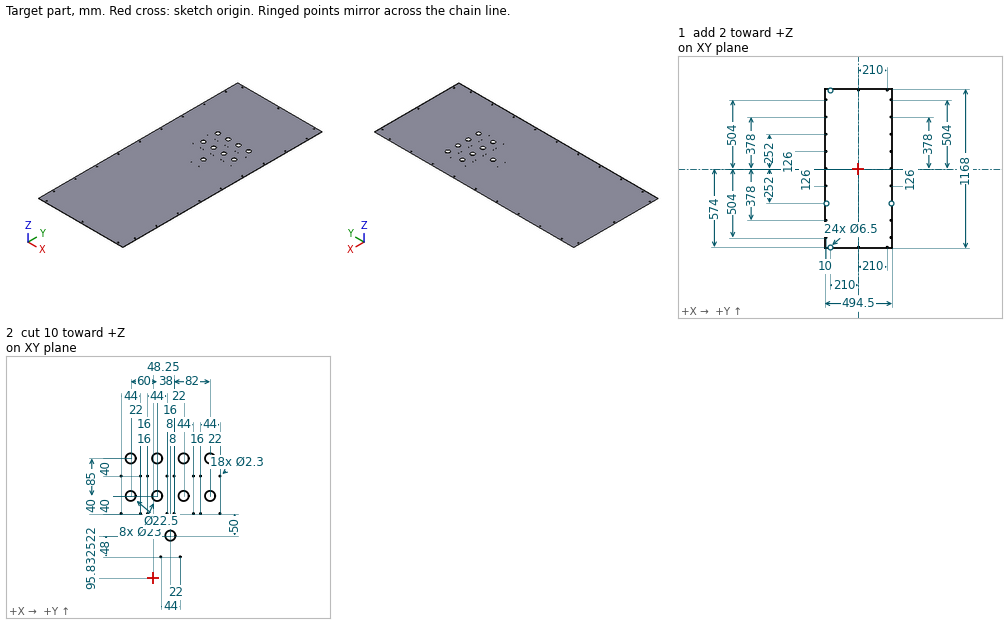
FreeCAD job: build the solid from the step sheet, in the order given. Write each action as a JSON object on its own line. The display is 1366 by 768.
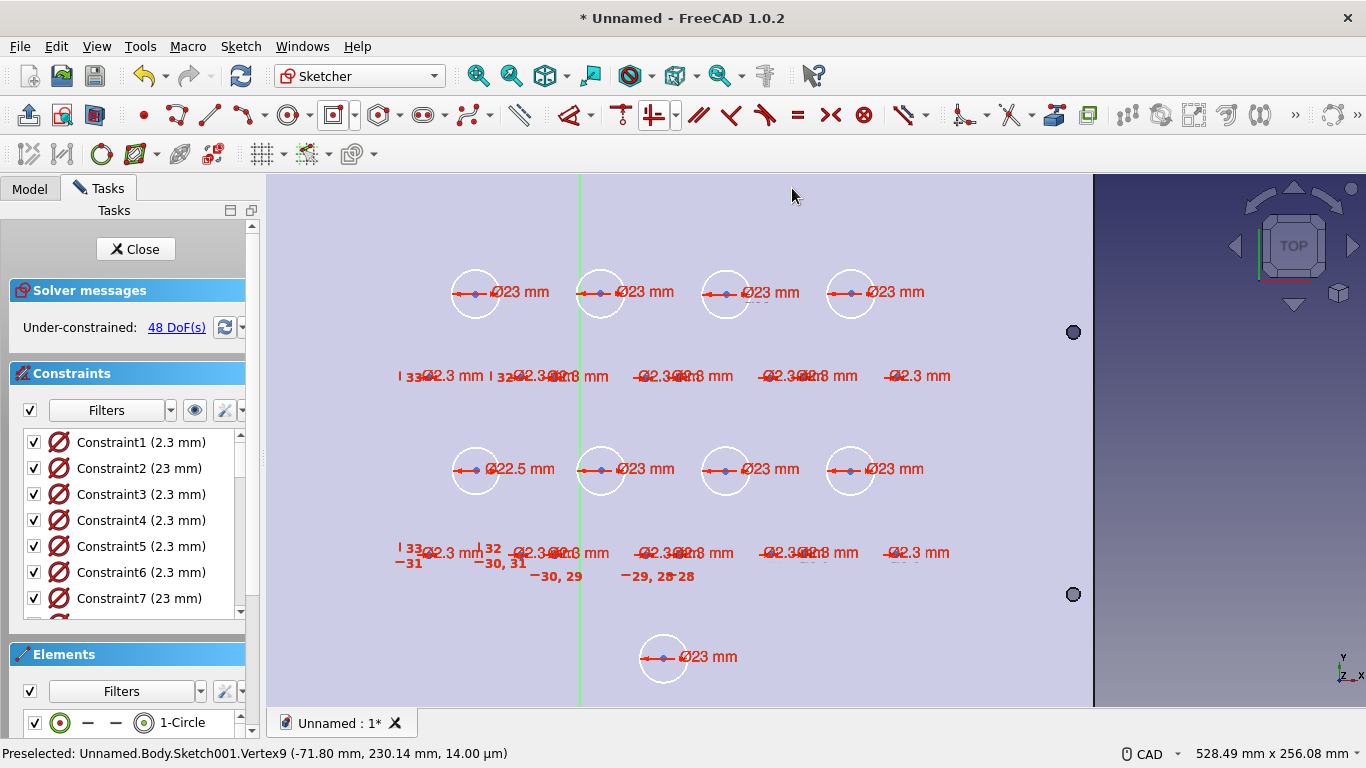
{"action": "left_click", "coordinate": [521, 378]}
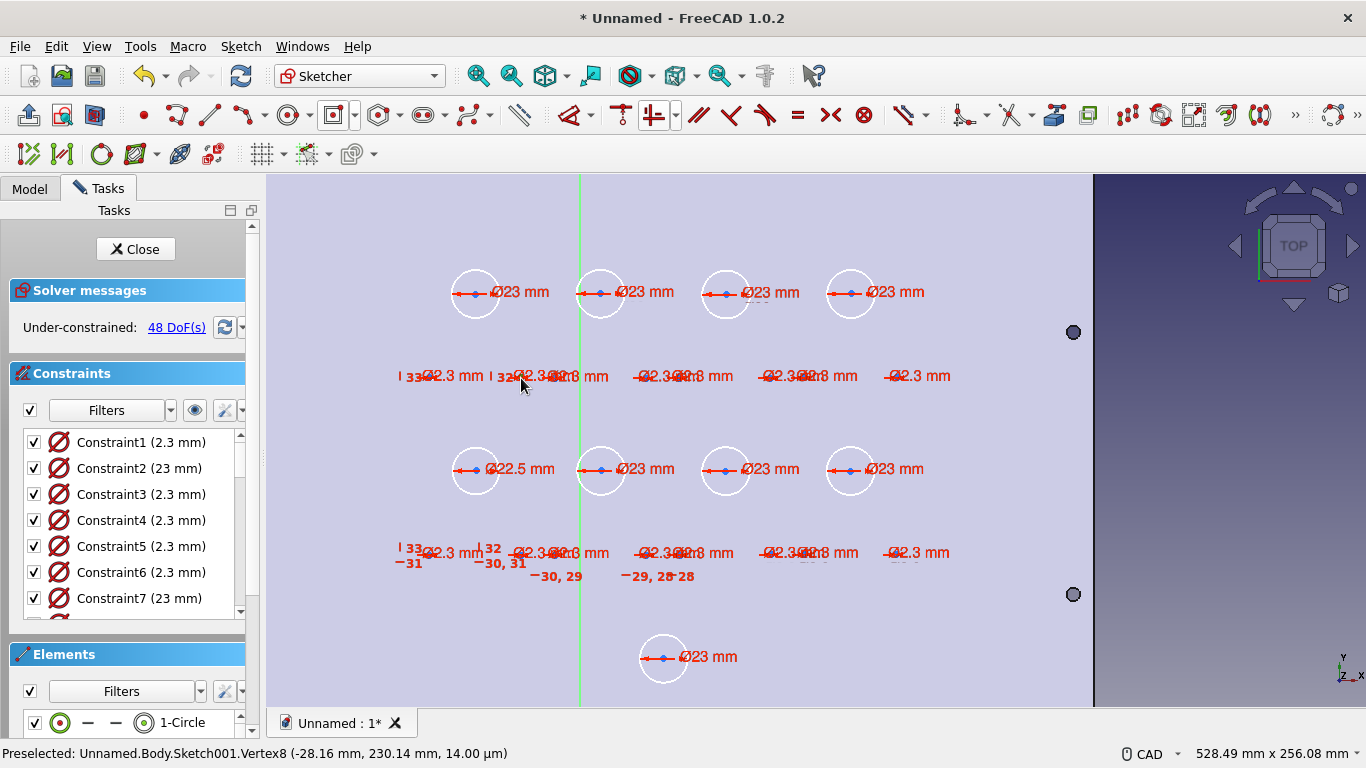
{"action": "left_click", "coordinate": [430, 378]}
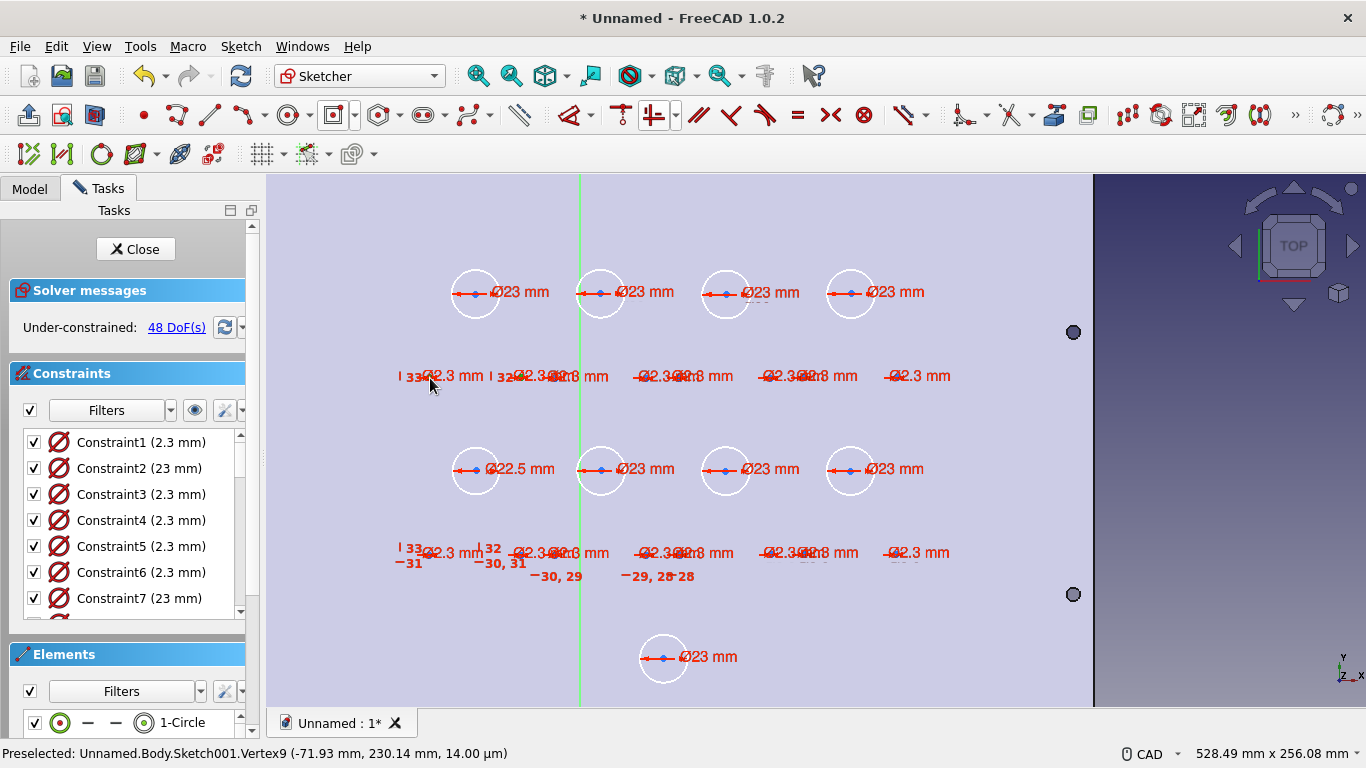
{"action": "left_click", "coordinate": [676, 116]}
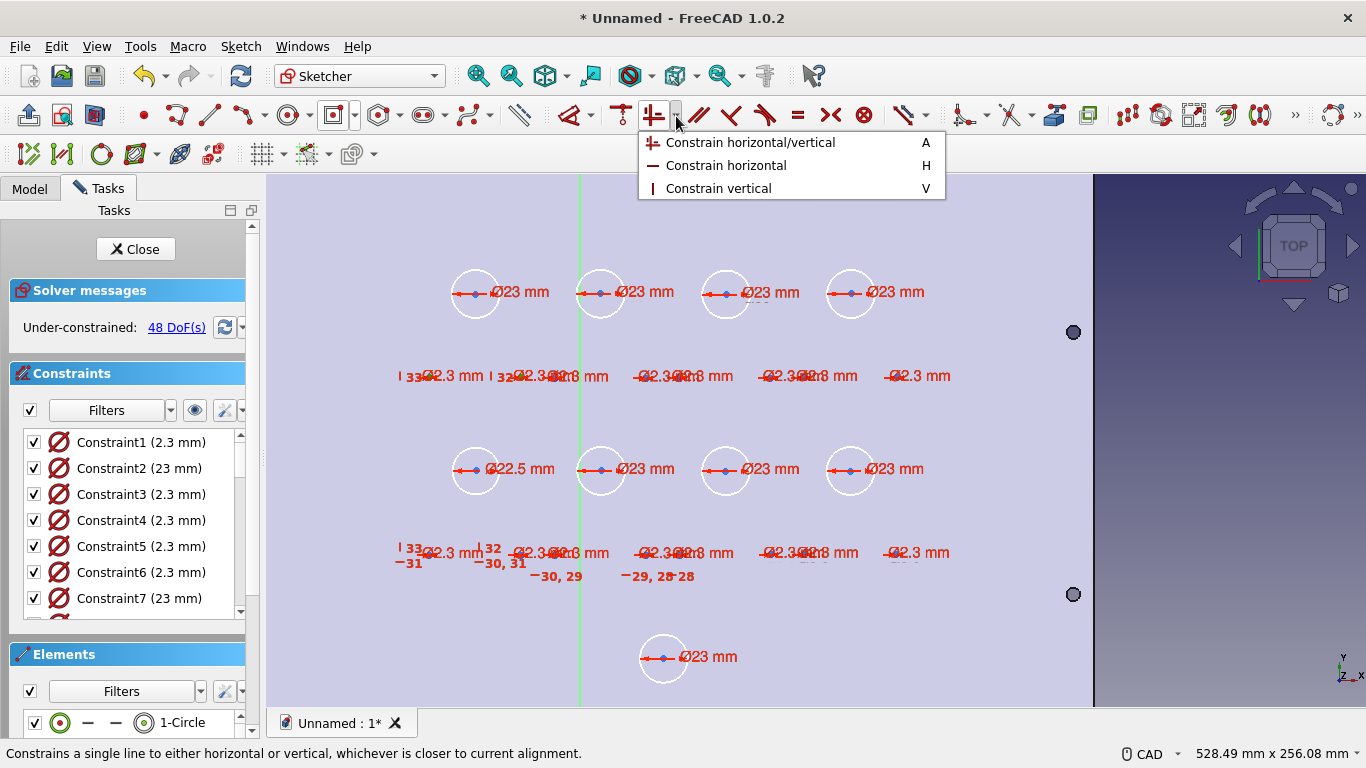
{"action": "left_click", "coordinate": [792, 166]}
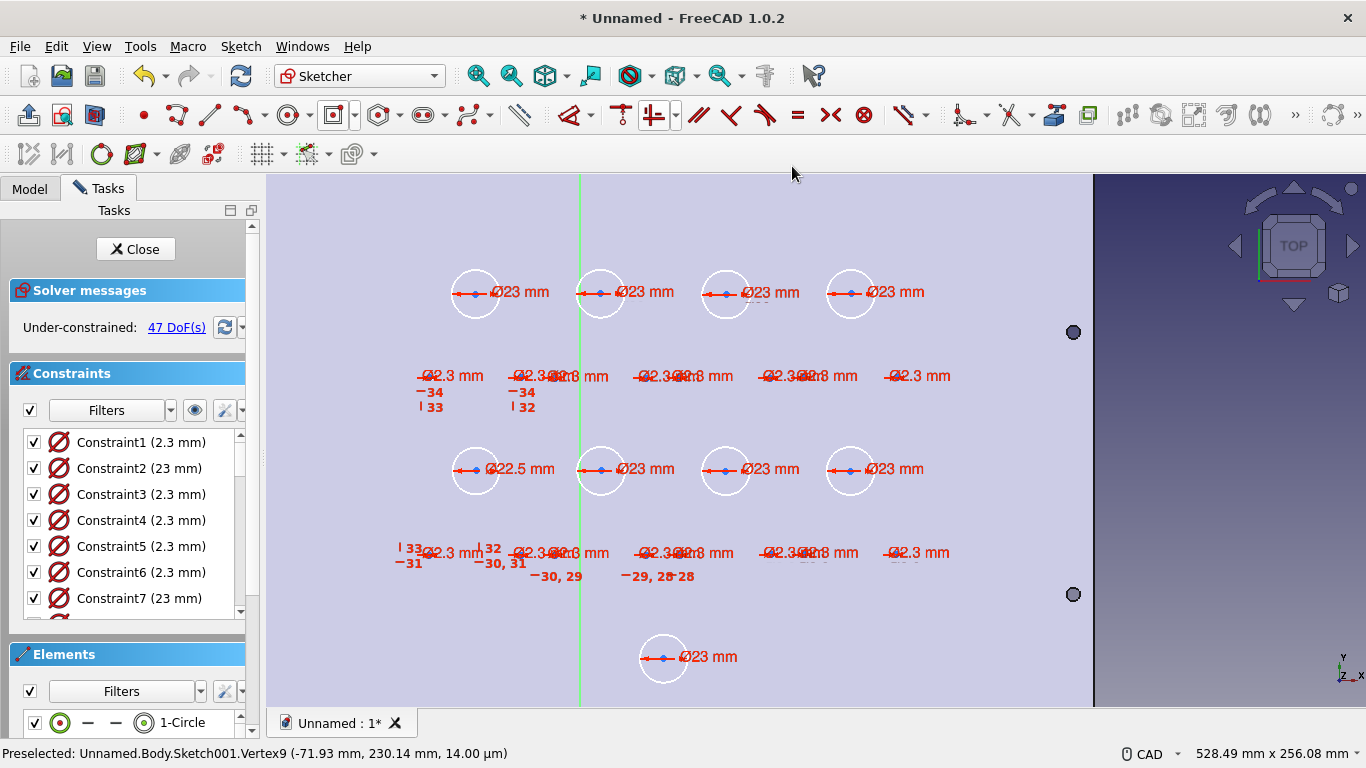
{"action": "left_click", "coordinate": [601, 471]}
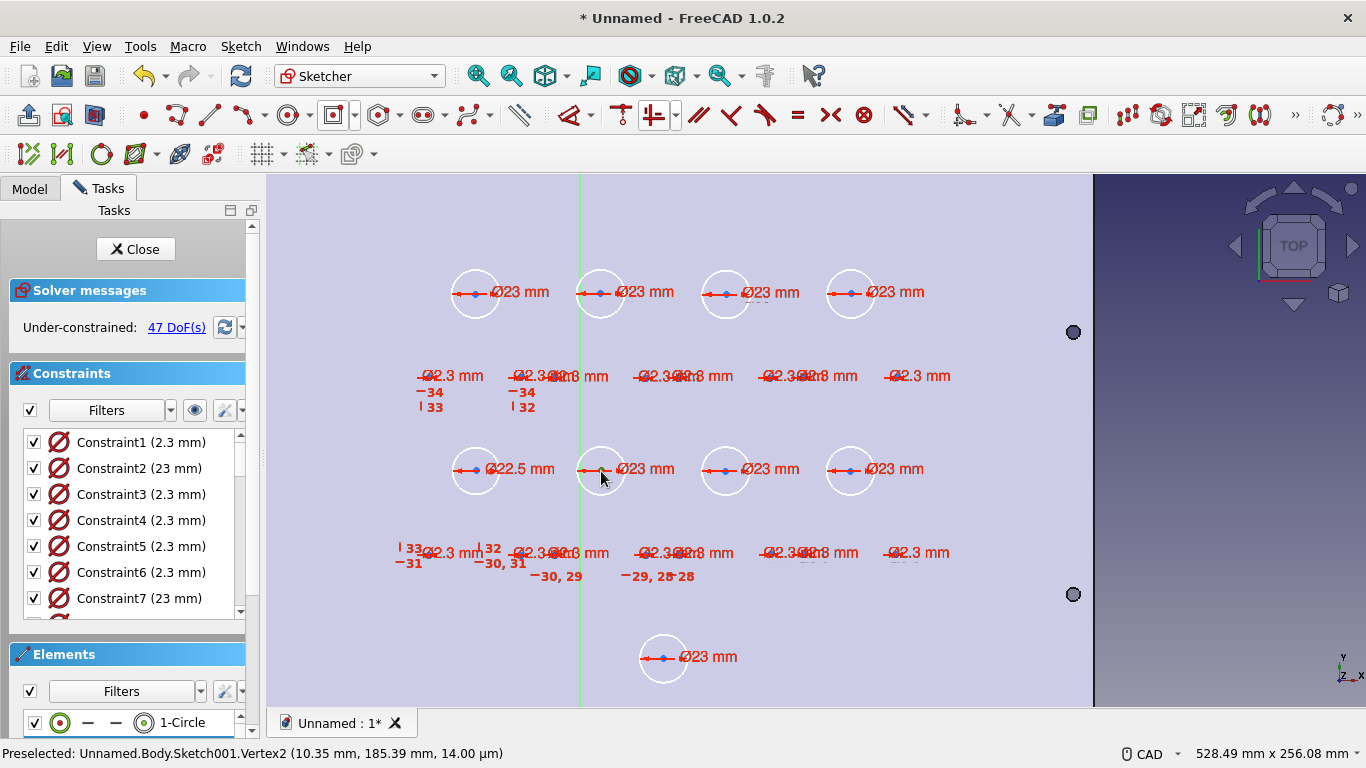
{"action": "left_click", "coordinate": [851, 471]}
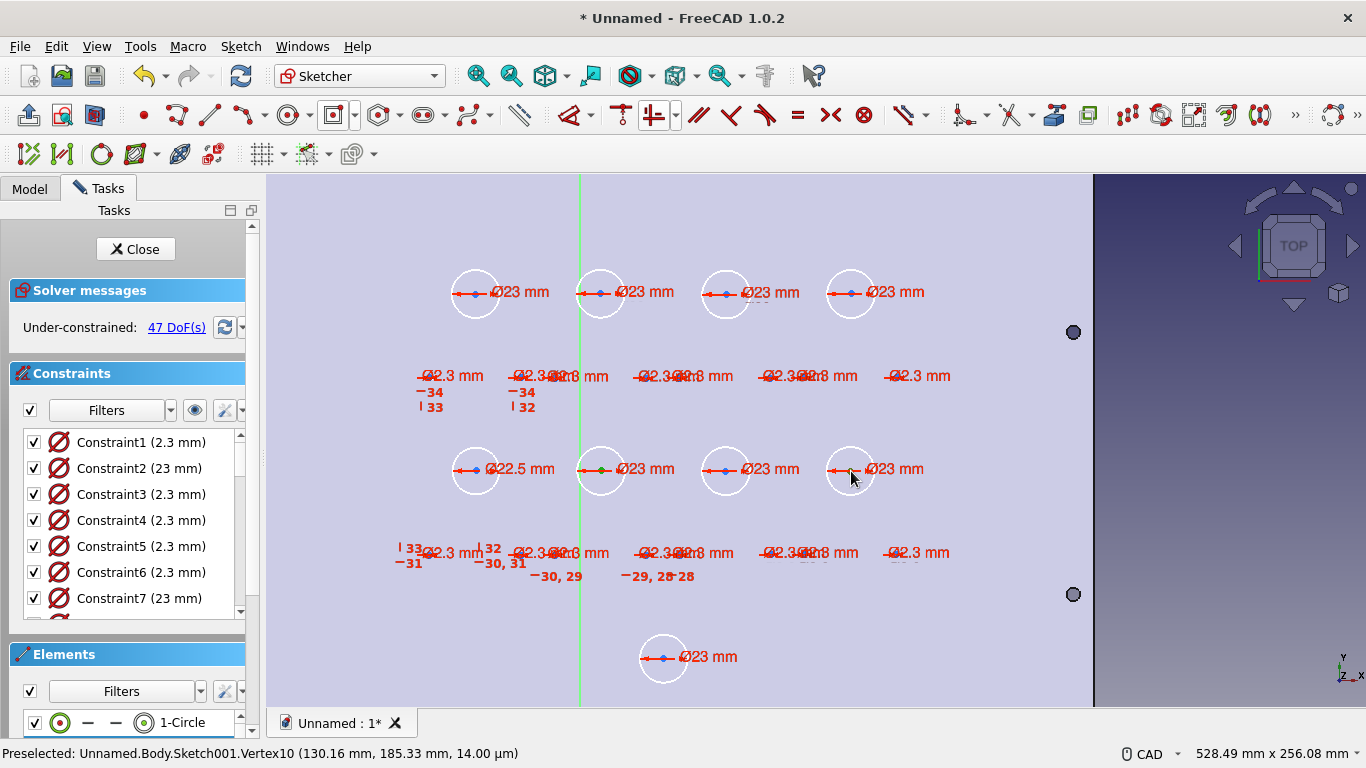
{"action": "left_click", "coordinate": [676, 116]}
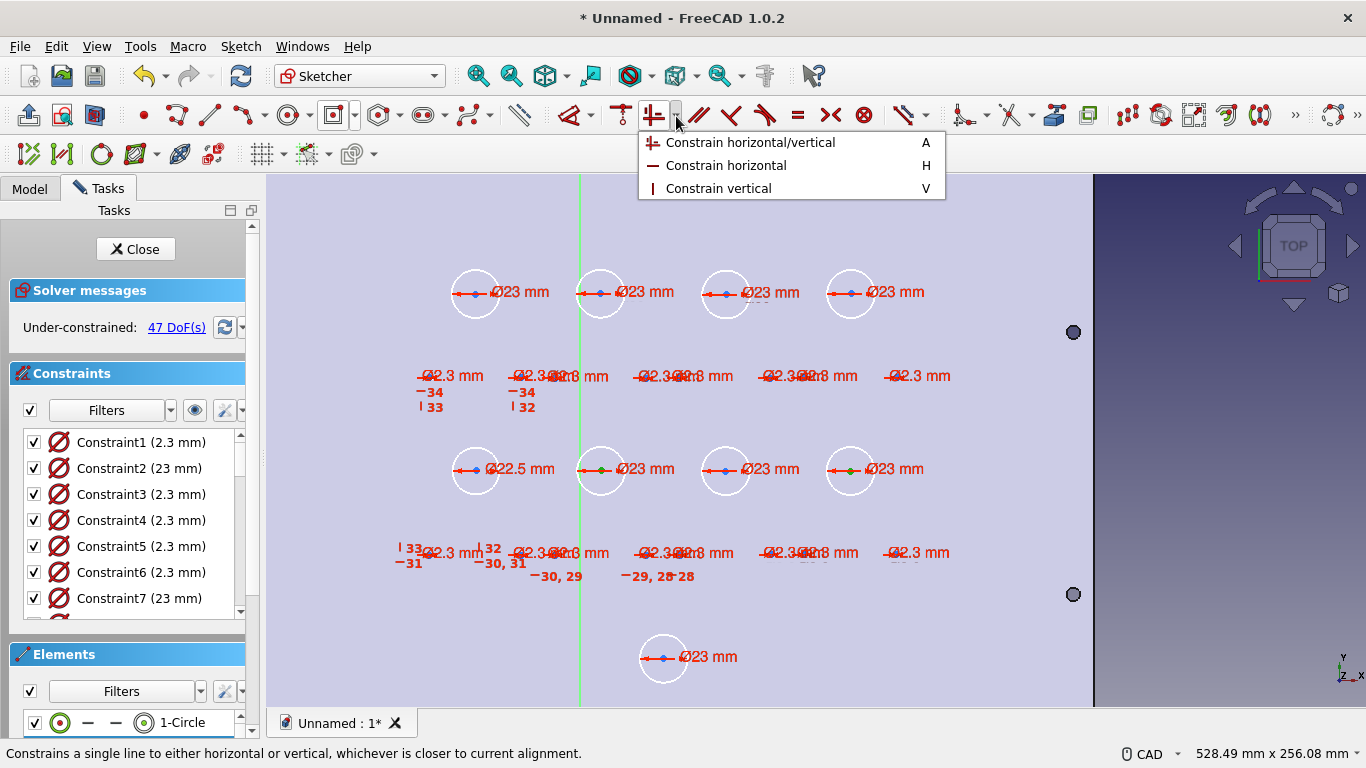
{"action": "left_click", "coordinate": [792, 166]}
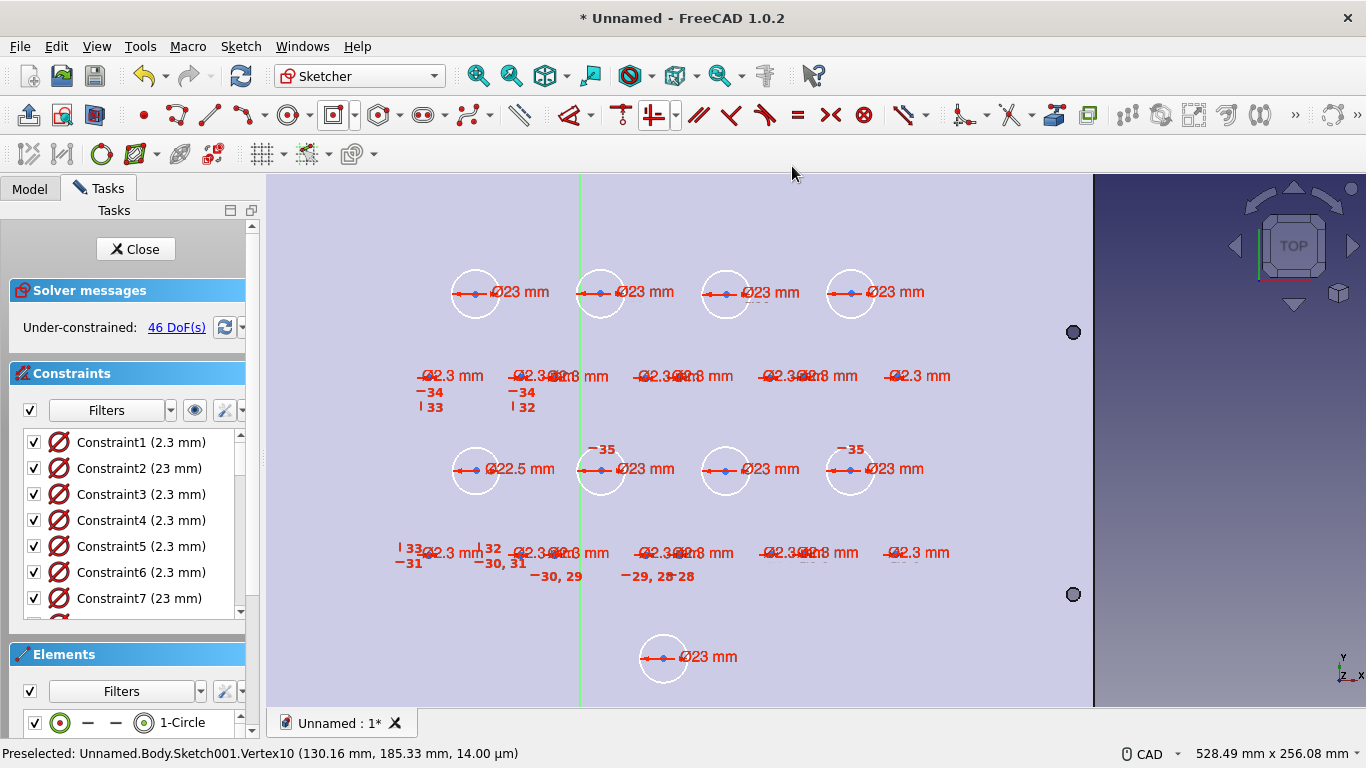
{"action": "left_click", "coordinate": [680, 555]}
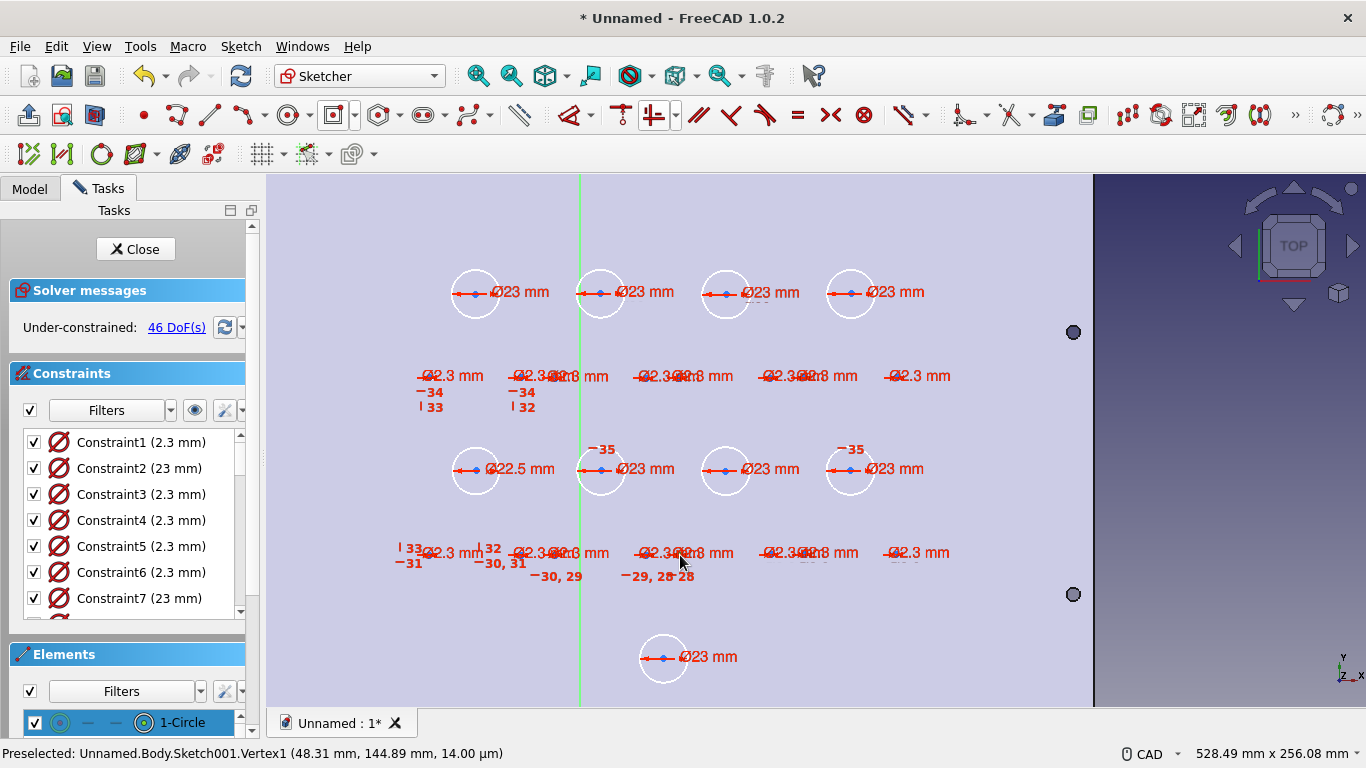
{"action": "left_click", "coordinate": [896, 555]}